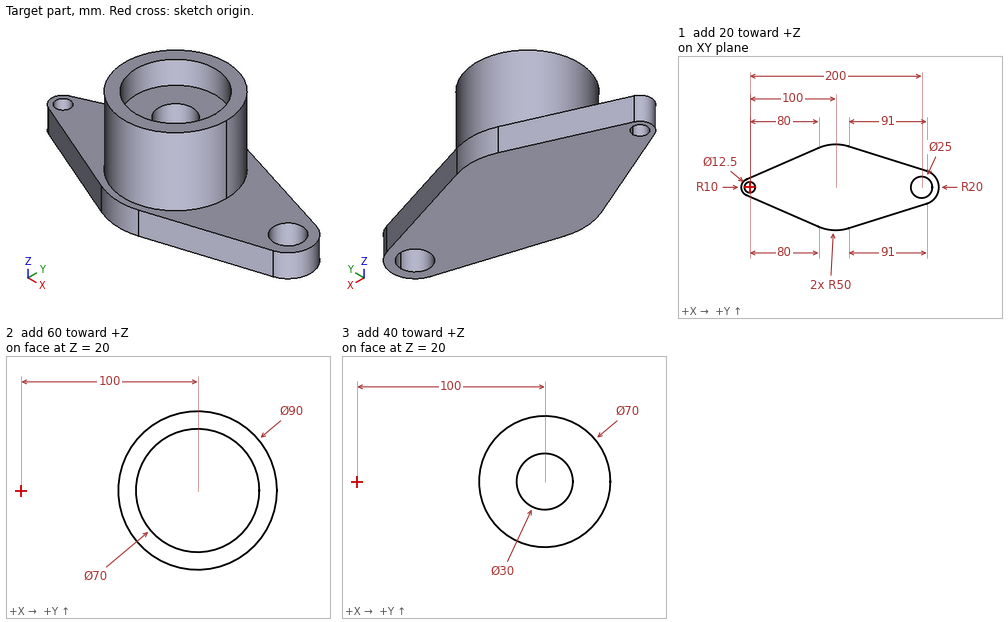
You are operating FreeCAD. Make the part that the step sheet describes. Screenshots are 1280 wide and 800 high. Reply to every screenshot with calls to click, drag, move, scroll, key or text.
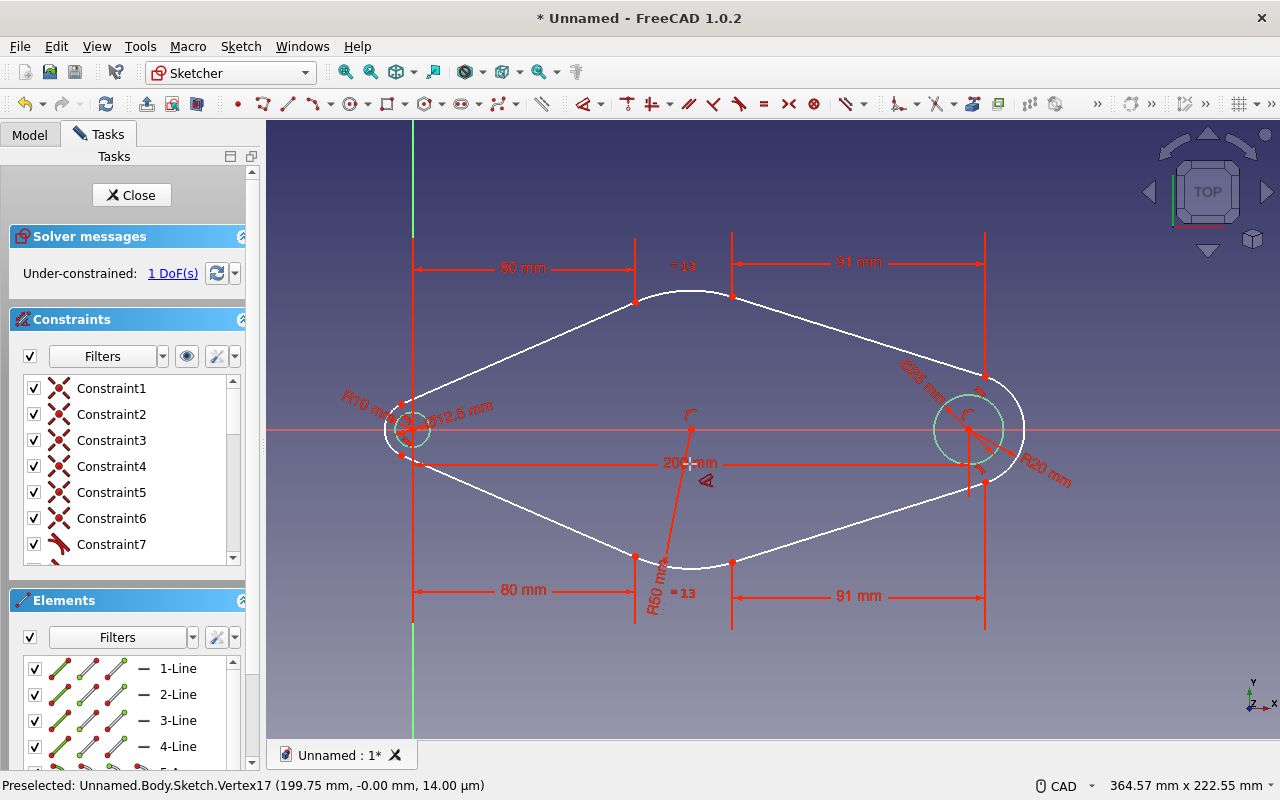
click(691, 430)
click(552, 464)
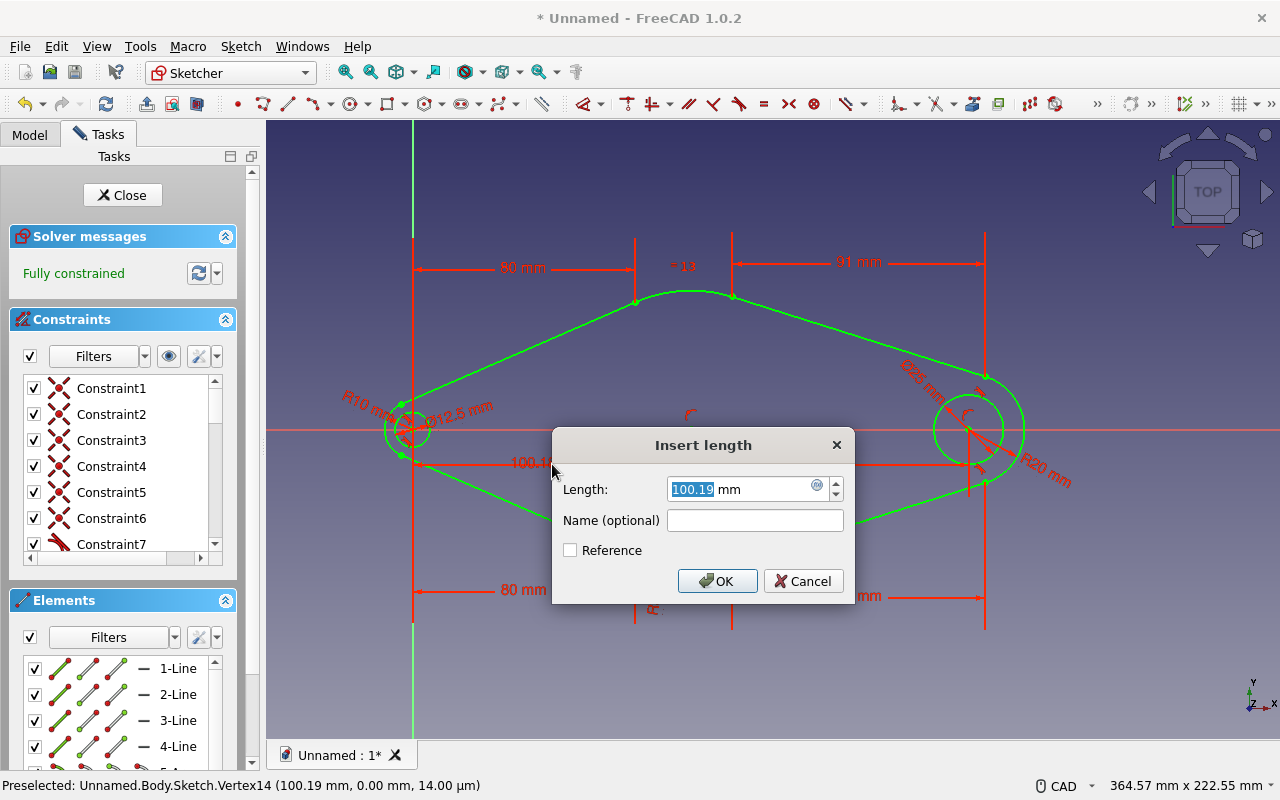
text(100)
key(Return)
key(Escape)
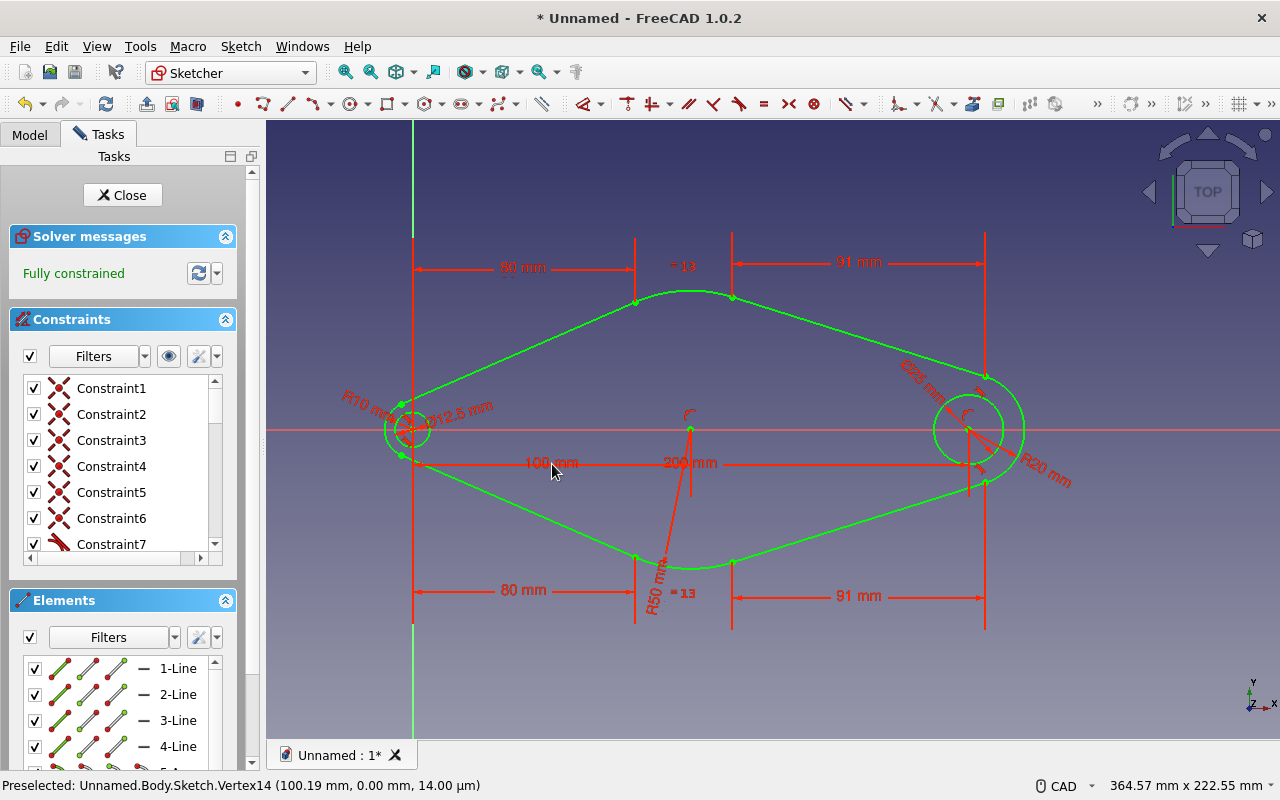
click(123, 195)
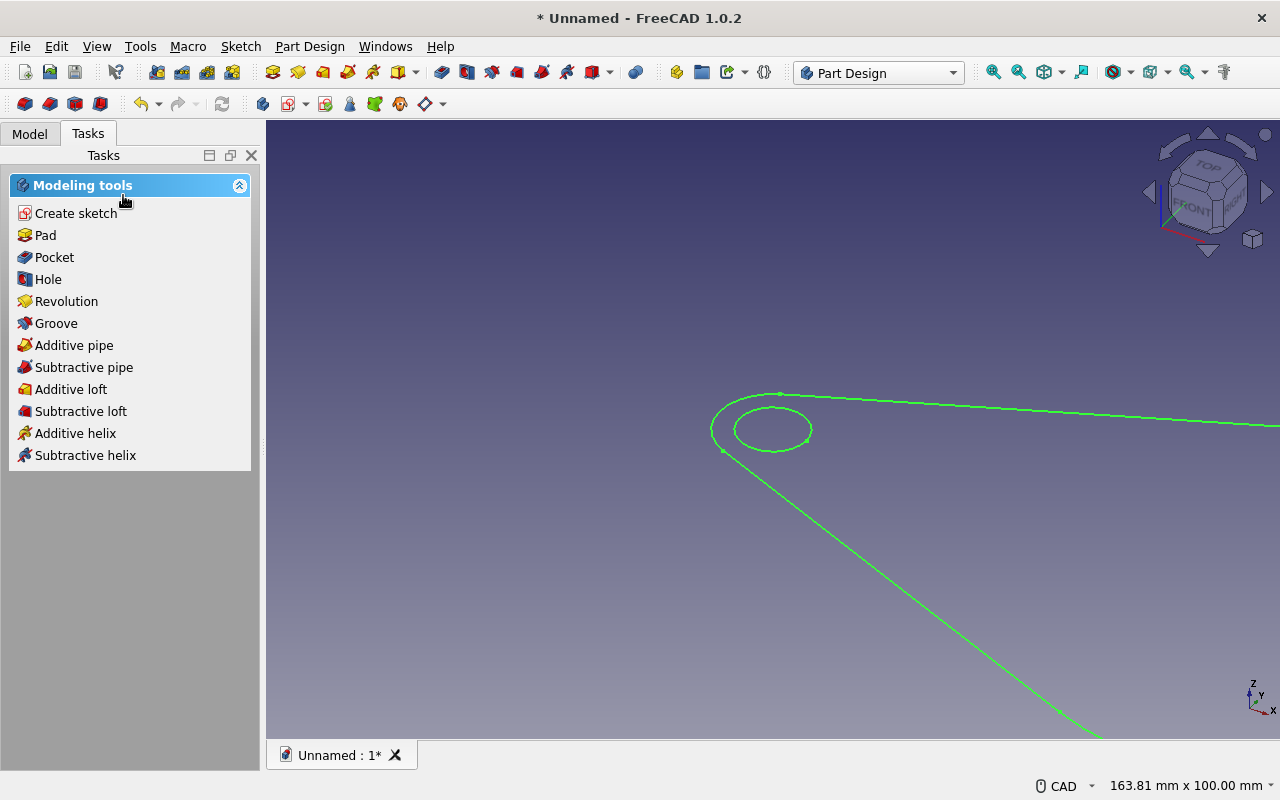
click(273, 72)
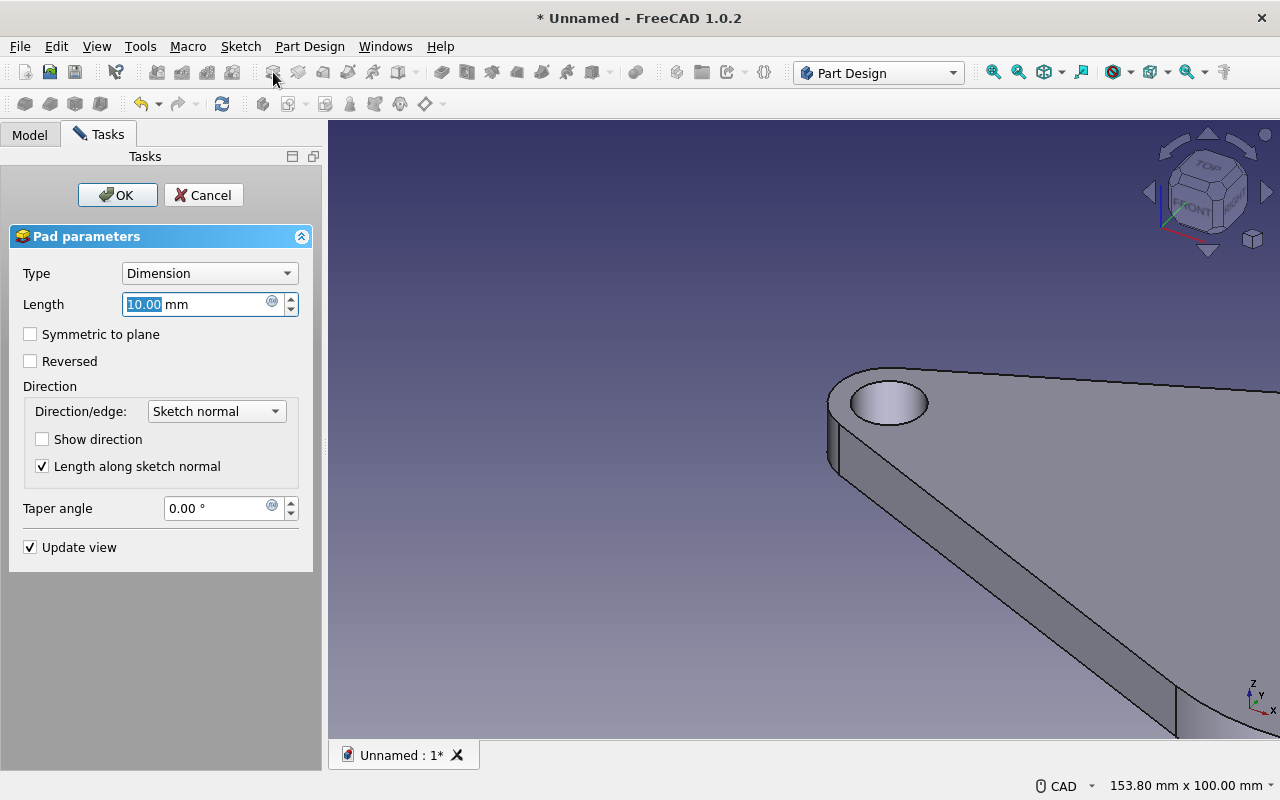
text(20)
key(Tab)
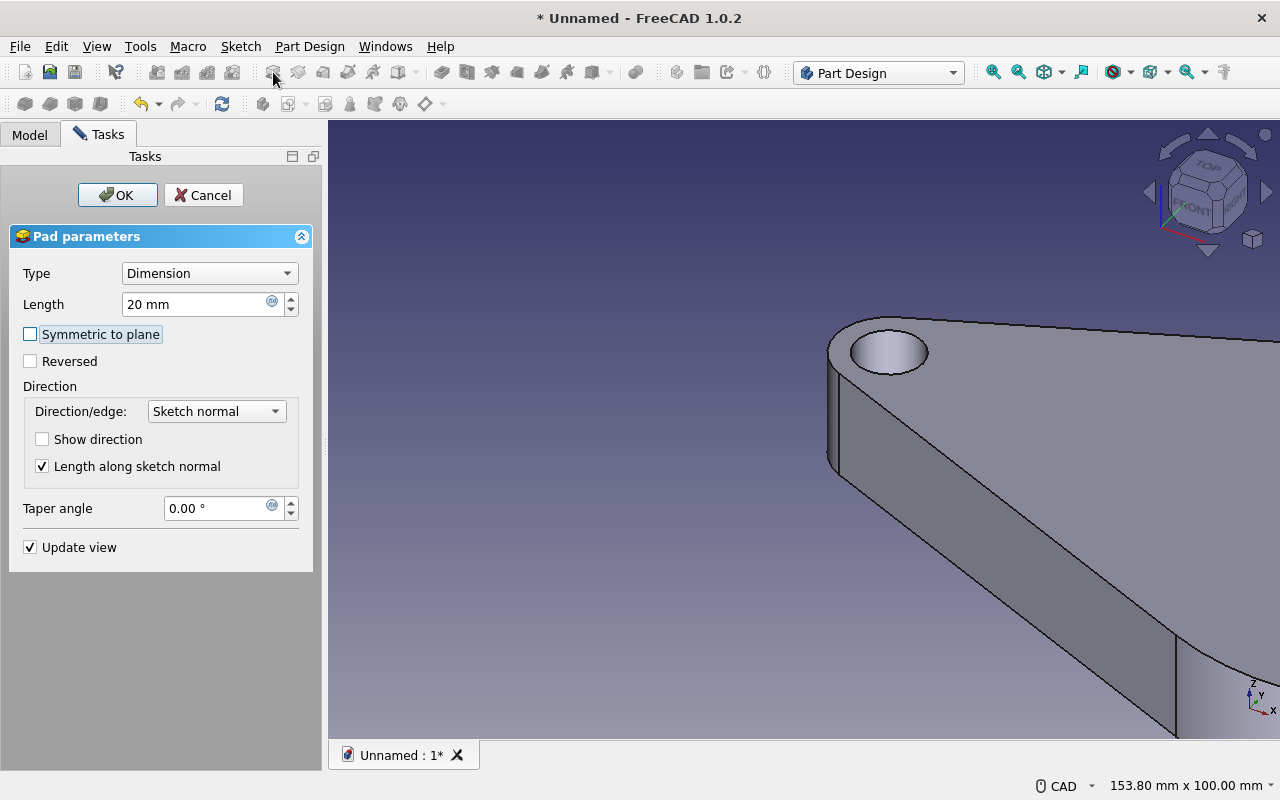
click(118, 195)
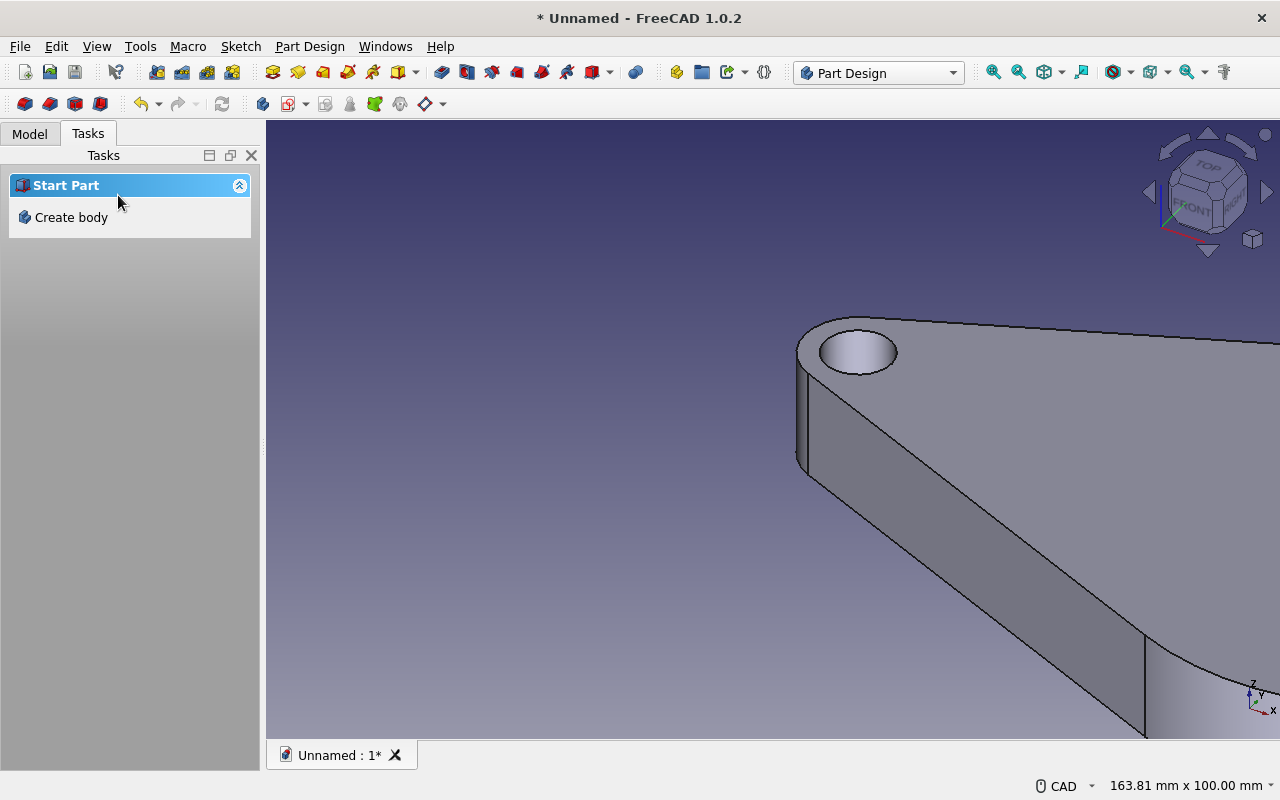
click(994, 72)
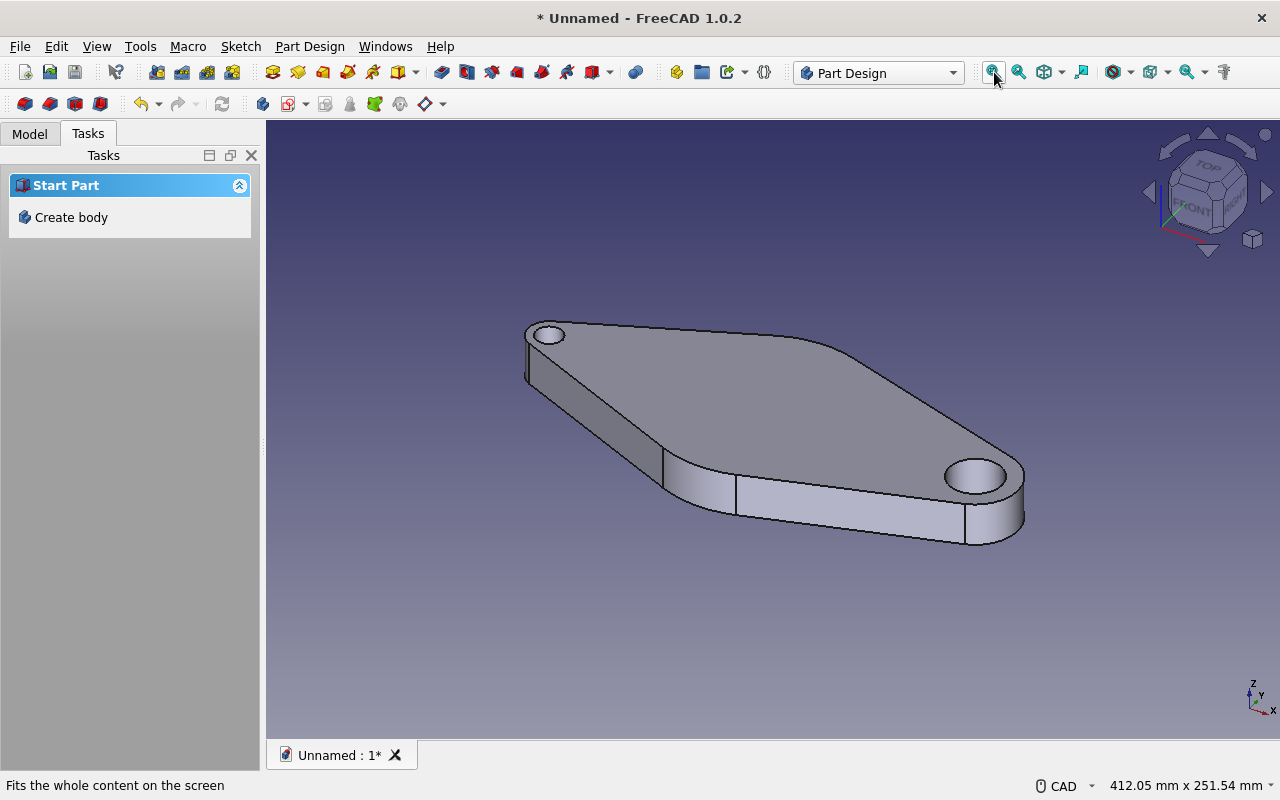
click(773, 408)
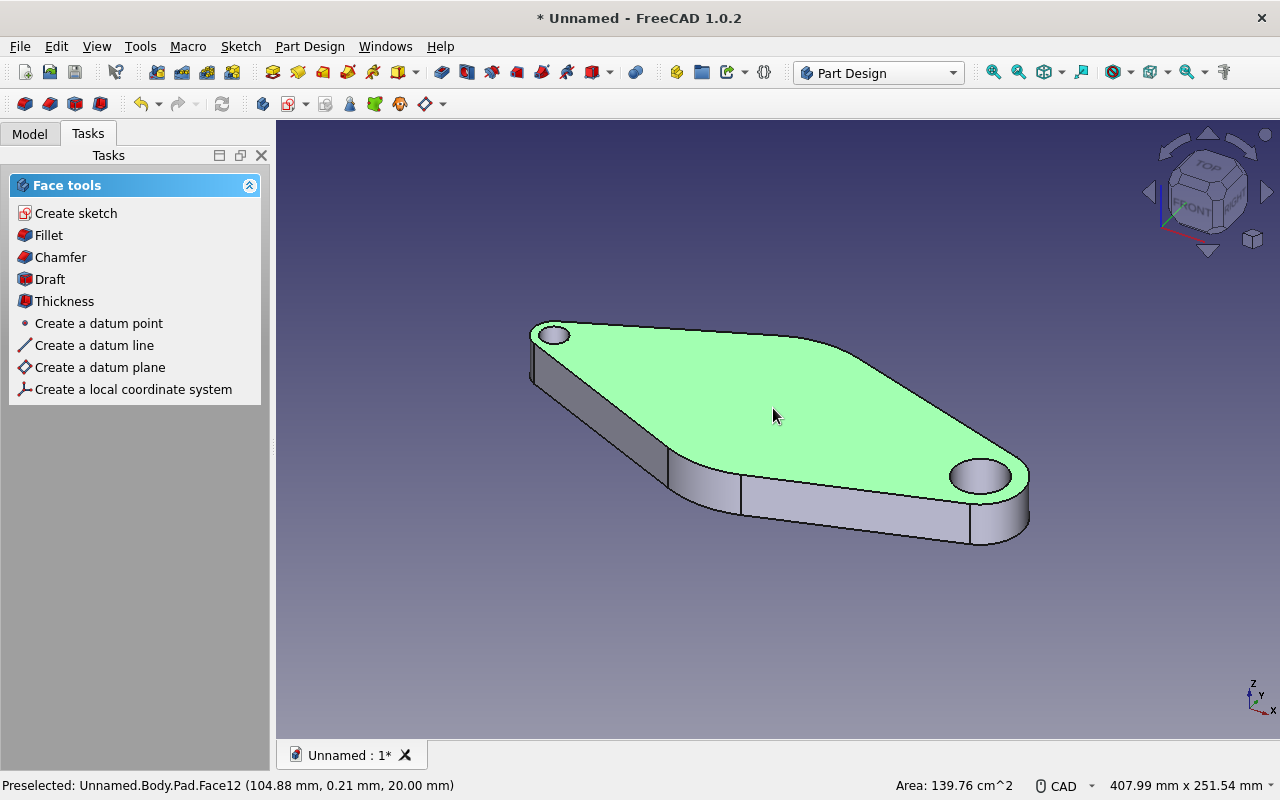
click(288, 104)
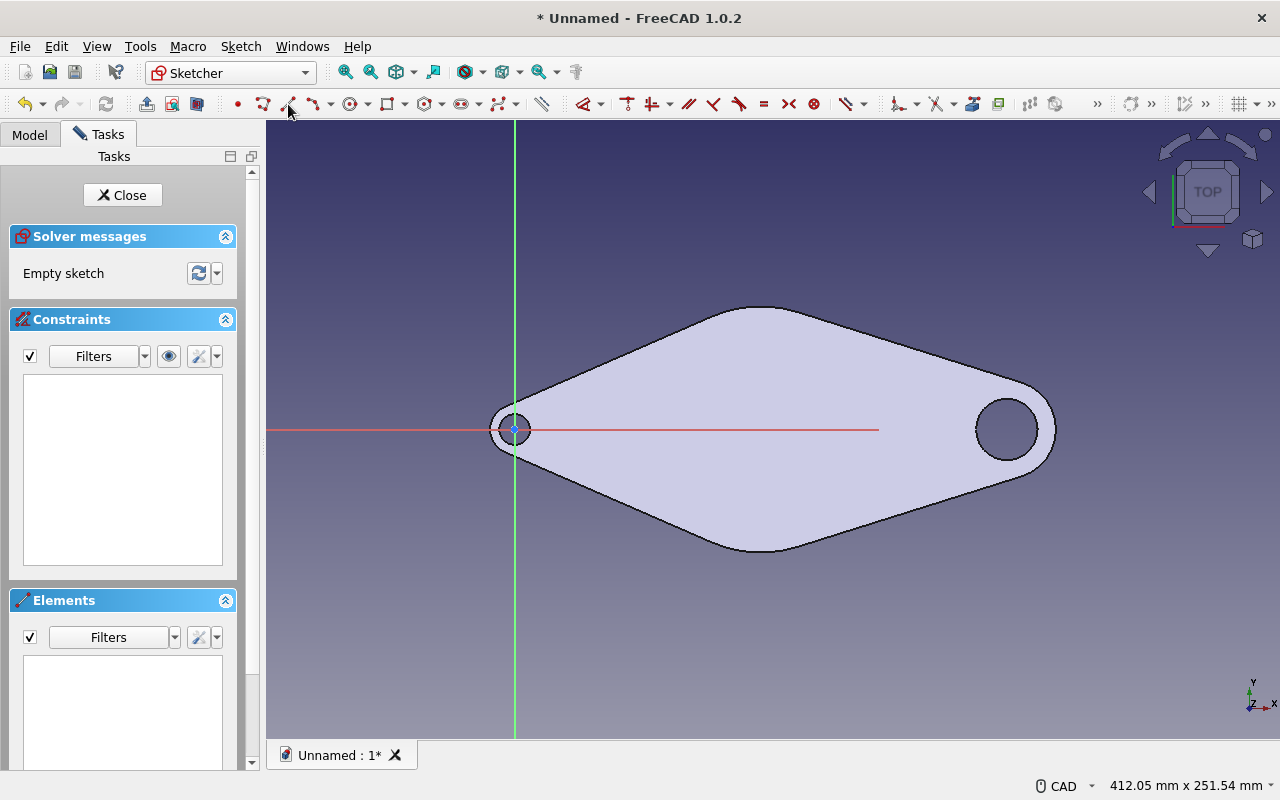
scroll(670, 429, up, 2)